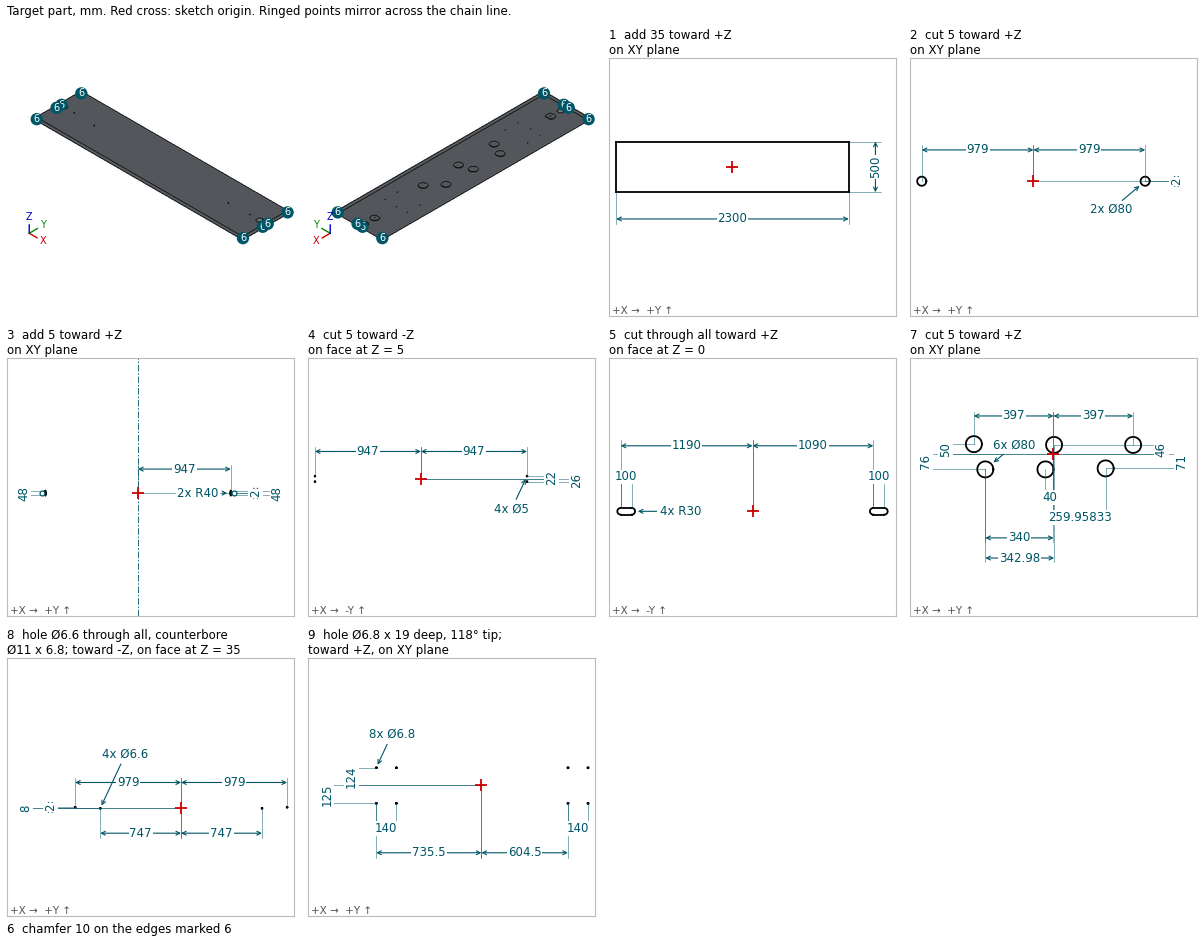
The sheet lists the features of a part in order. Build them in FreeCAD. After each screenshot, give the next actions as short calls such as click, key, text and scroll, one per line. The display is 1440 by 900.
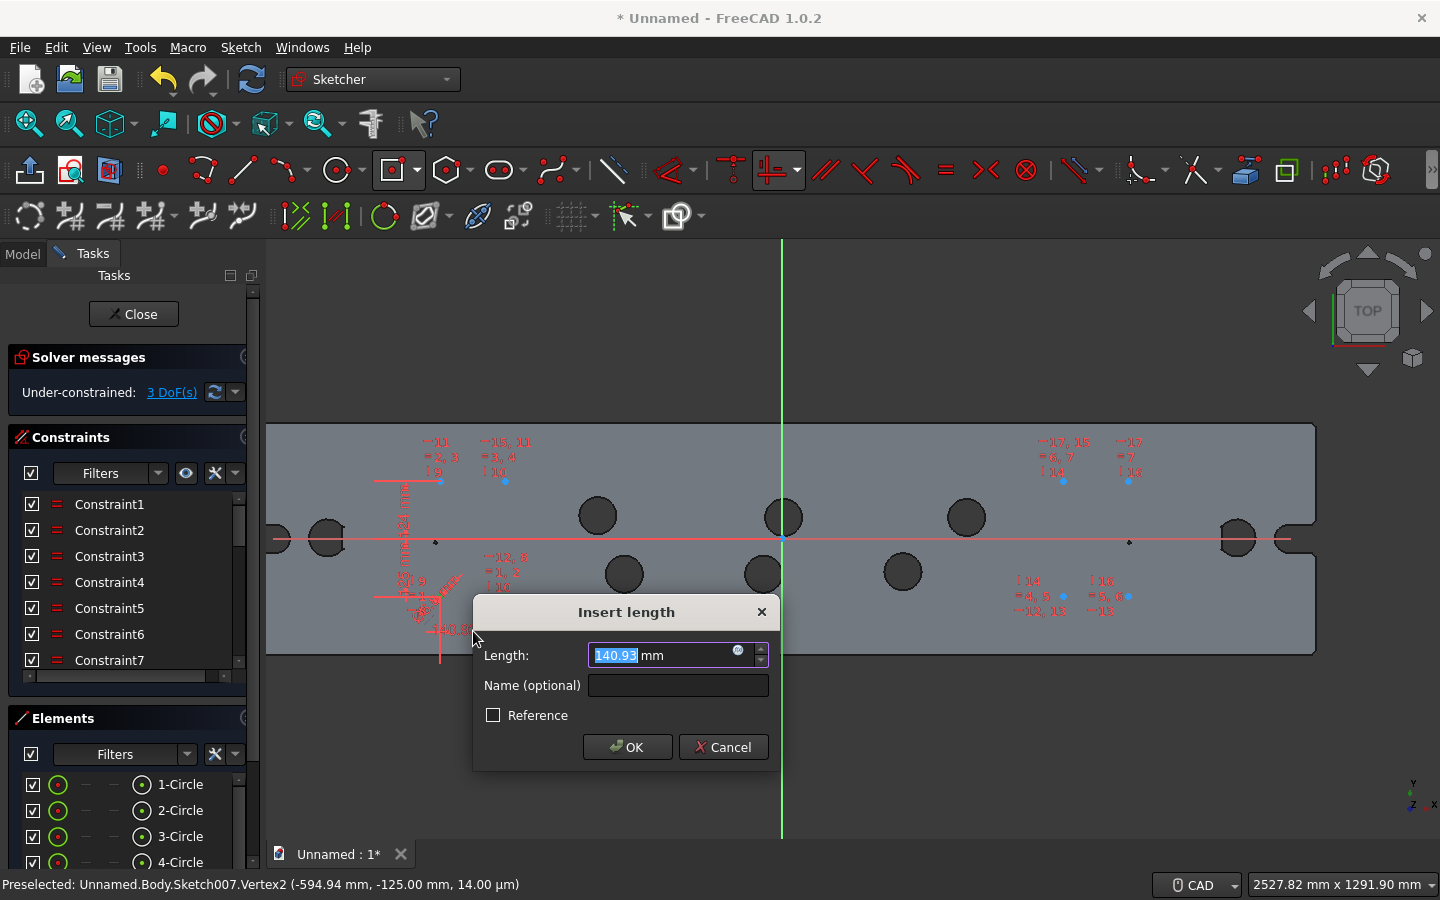
text(140)
key(Return)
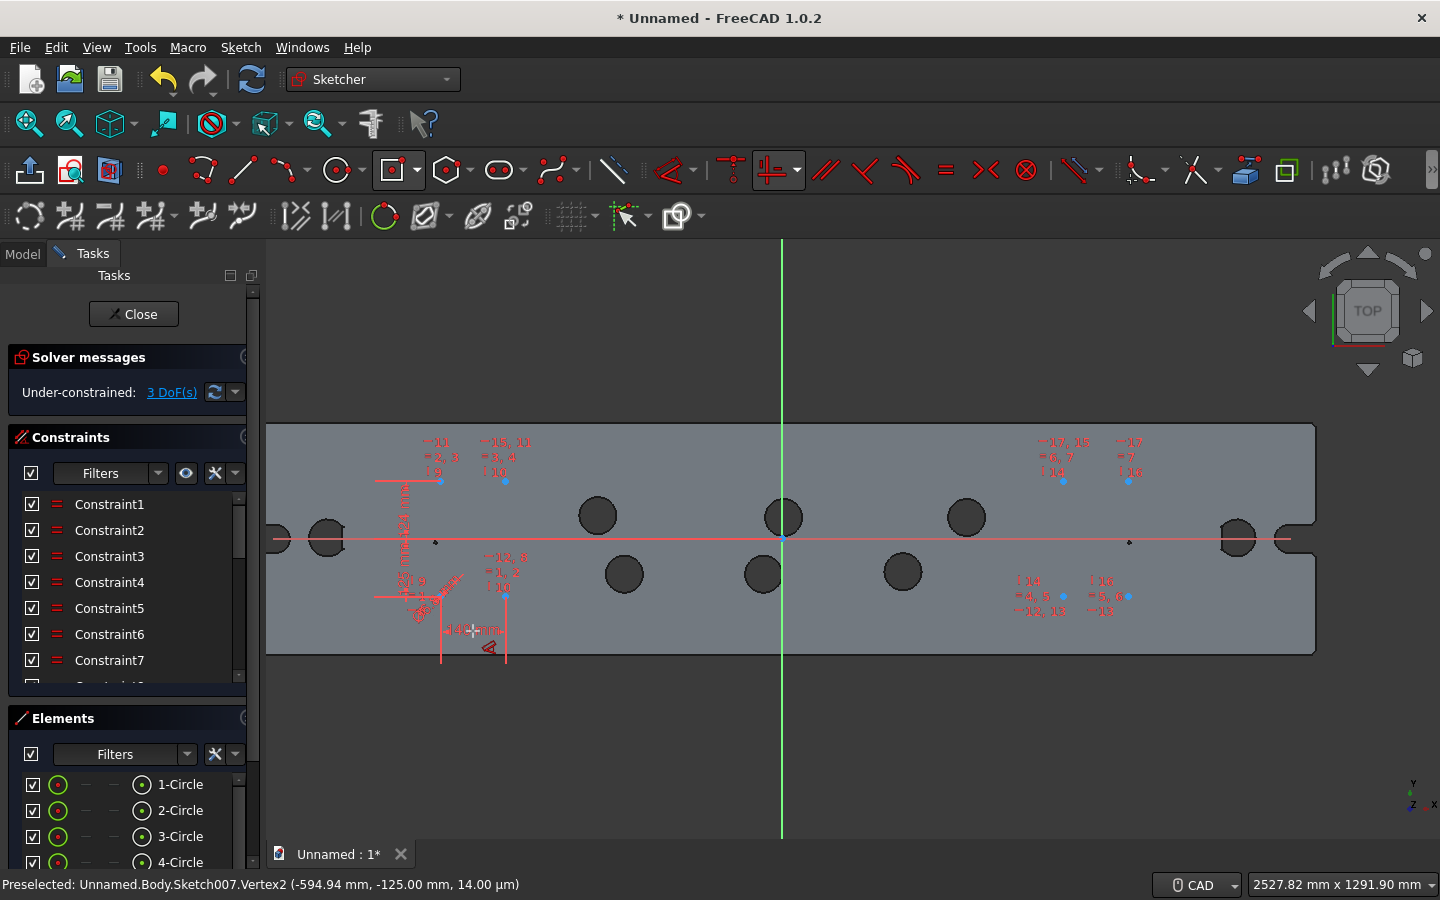
click(1063, 597)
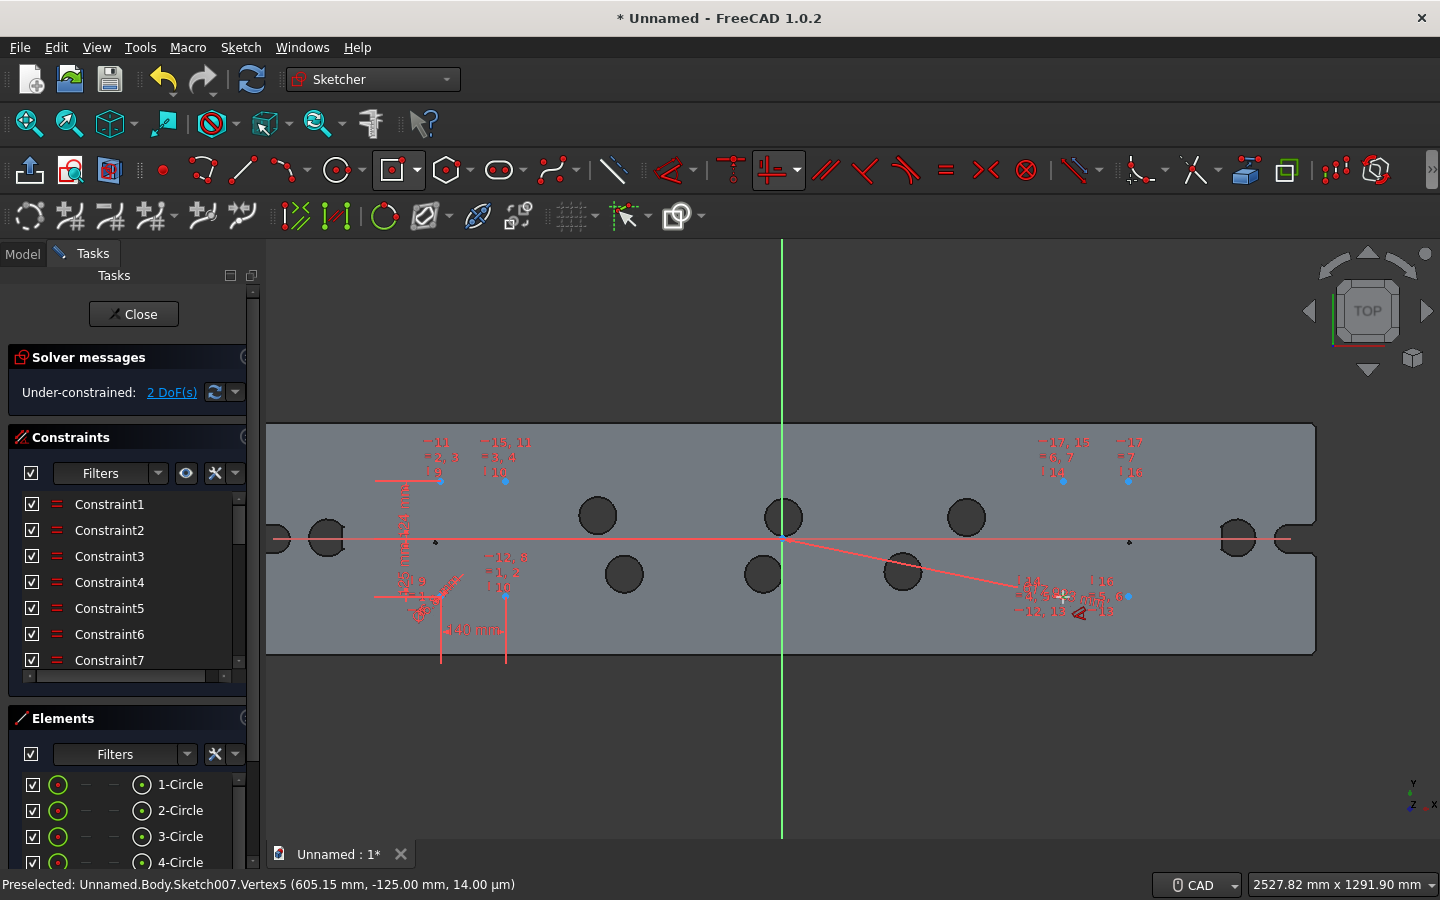
click(1128, 597)
click(1096, 631)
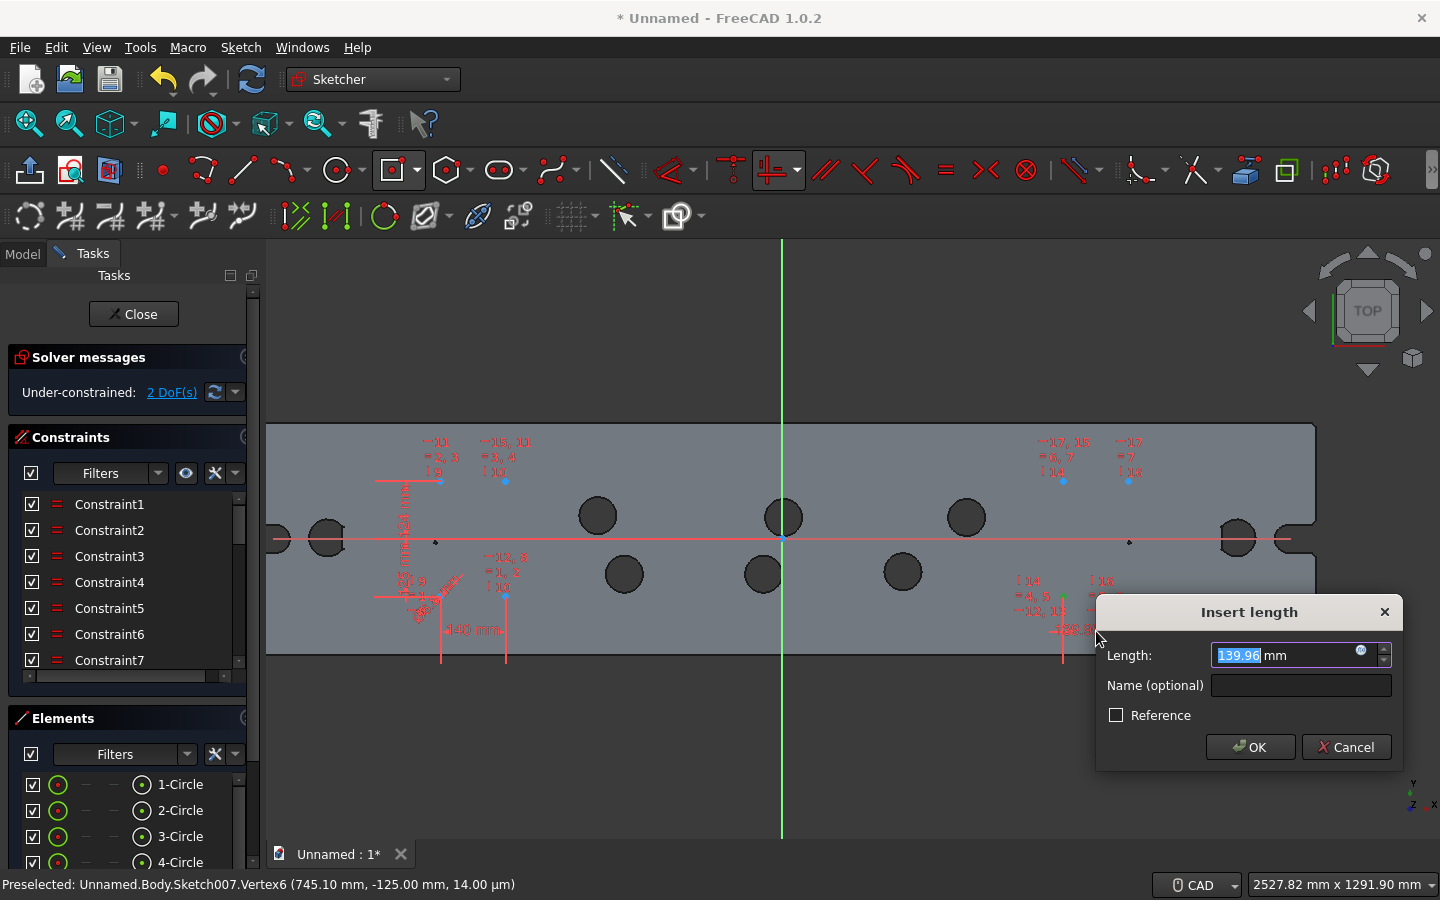
text(140)
key(Return)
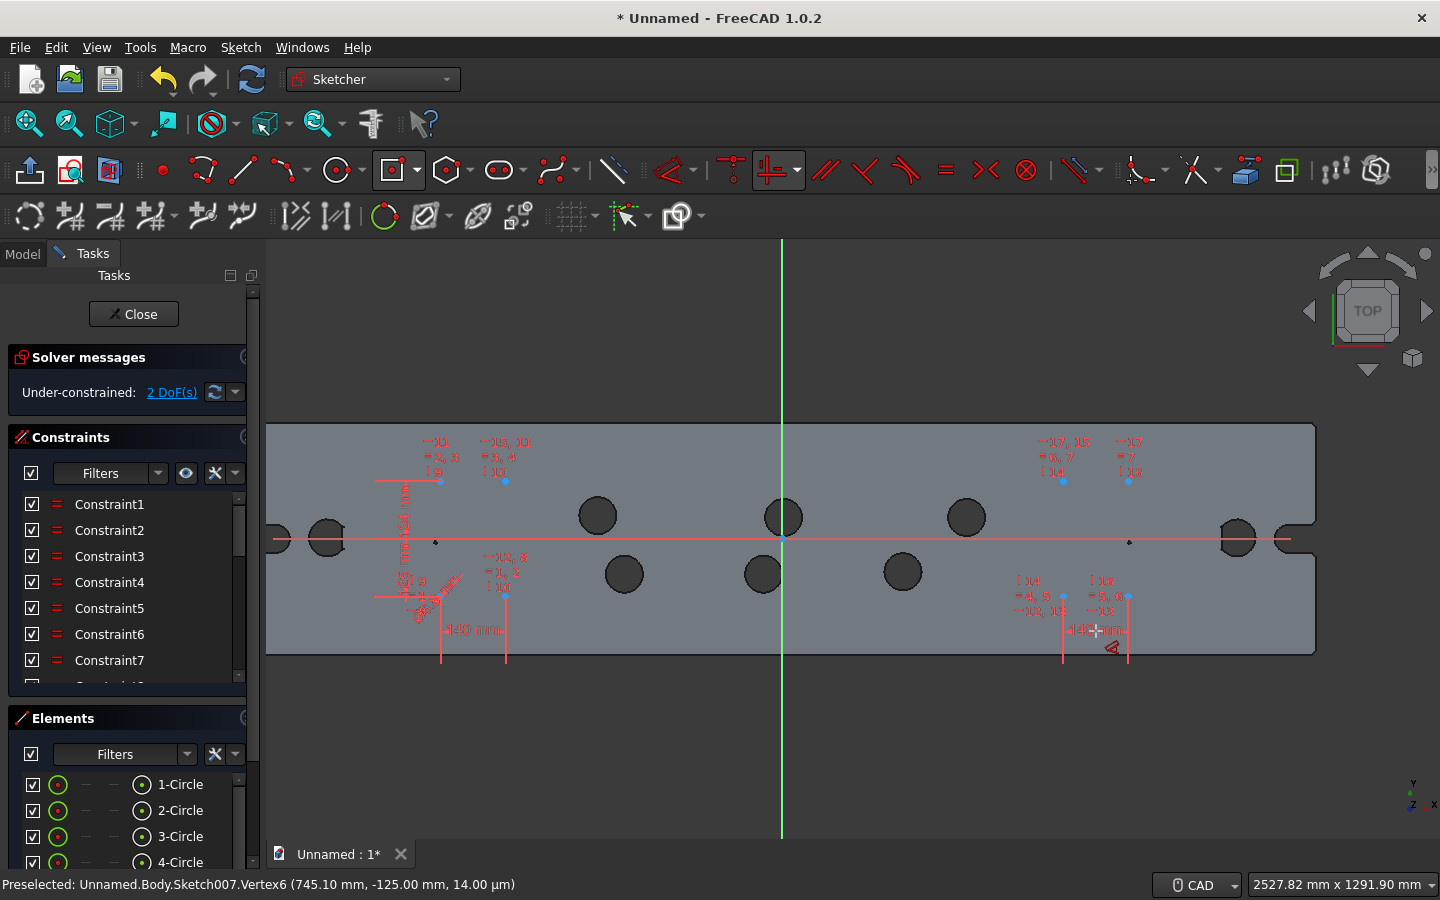
click(441, 597)
click(612, 631)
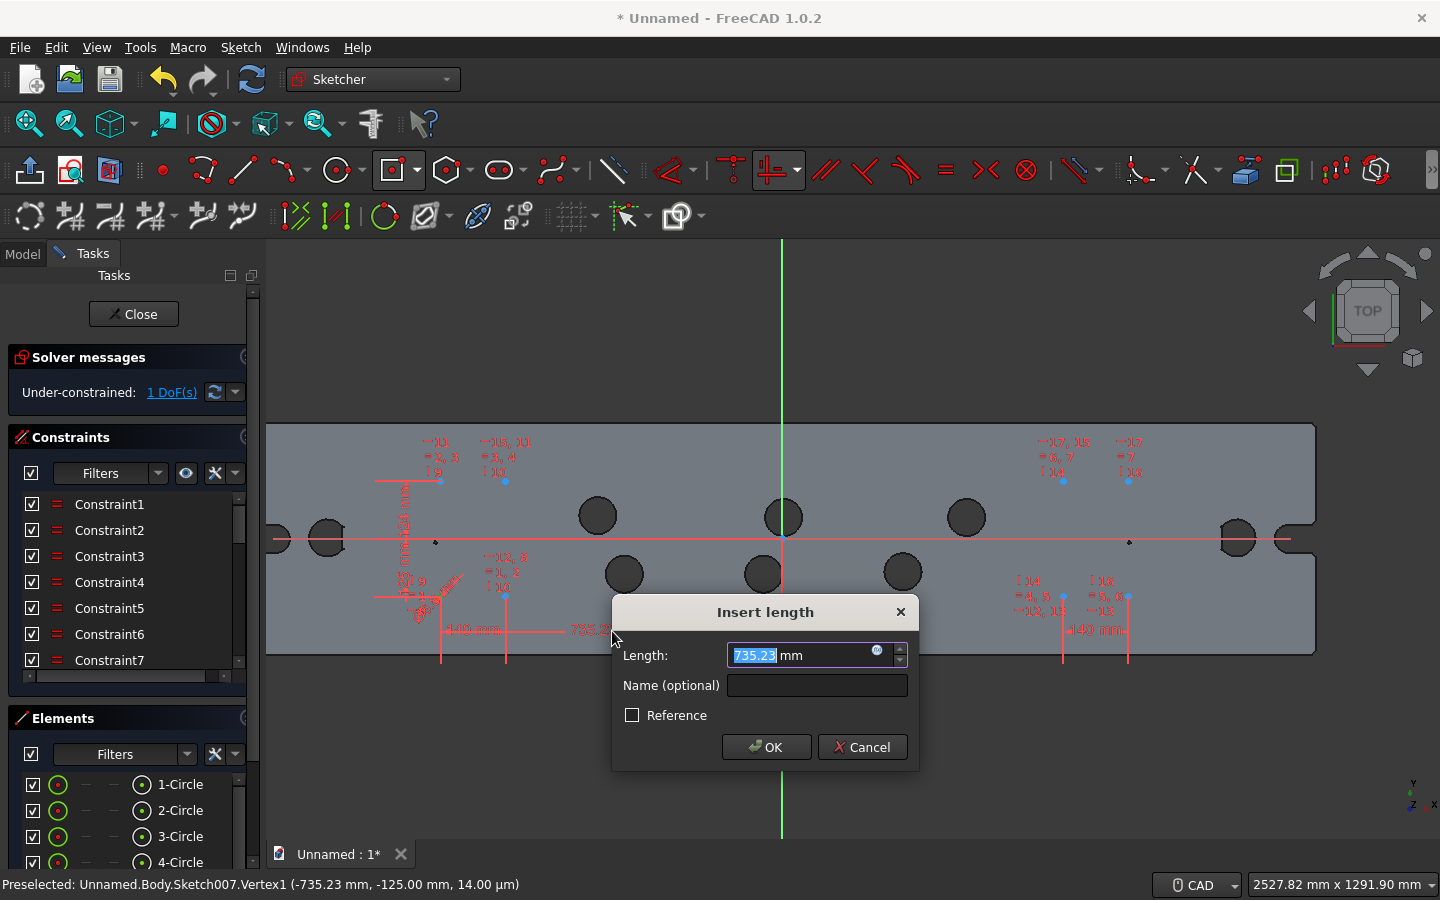
text(735.5)
key(Return)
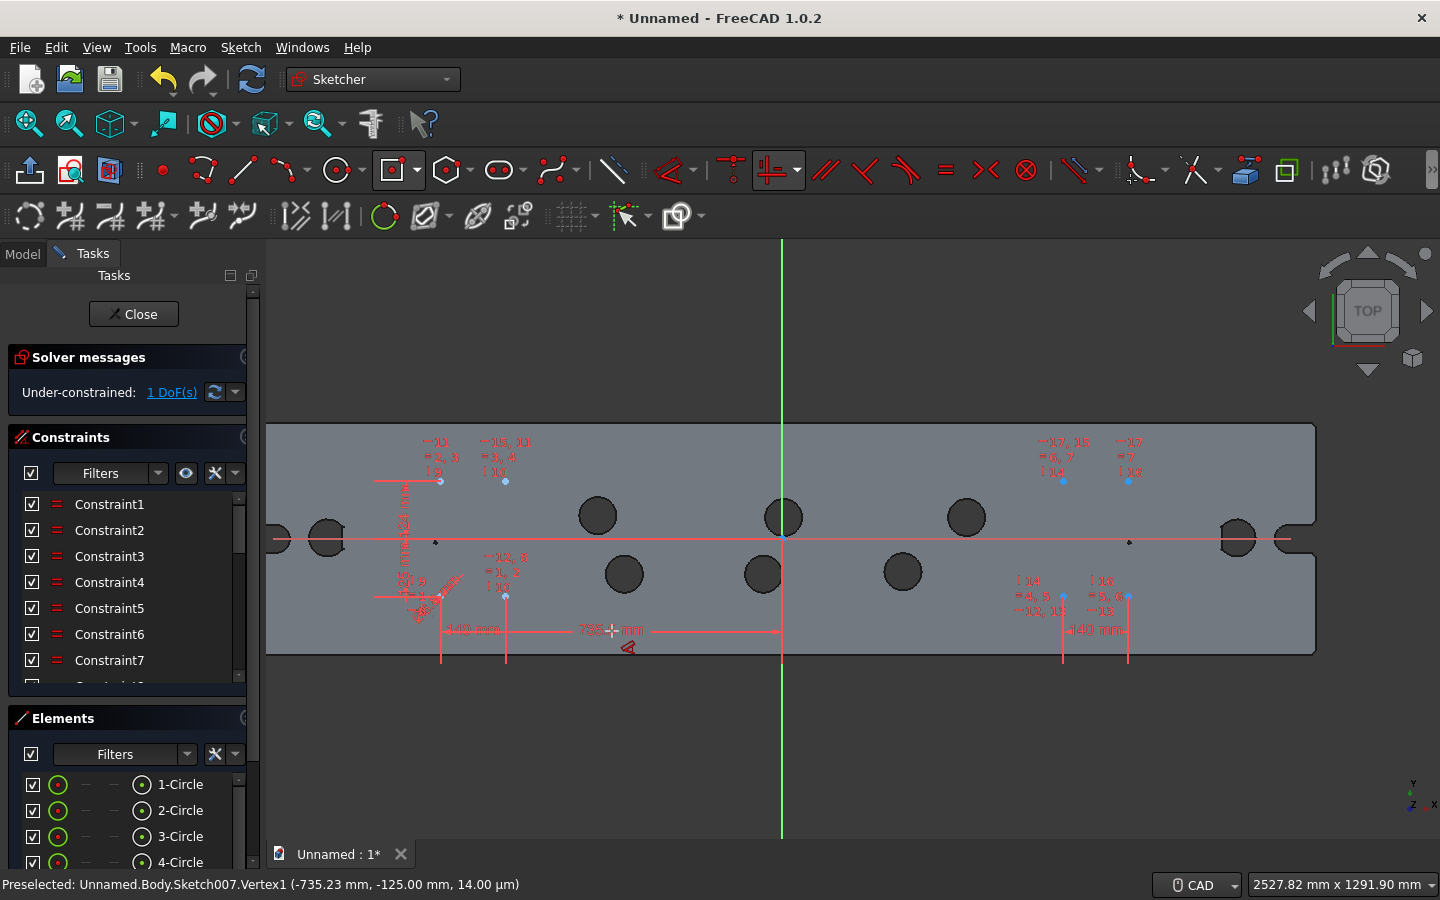
click(1063, 597)
click(923, 631)